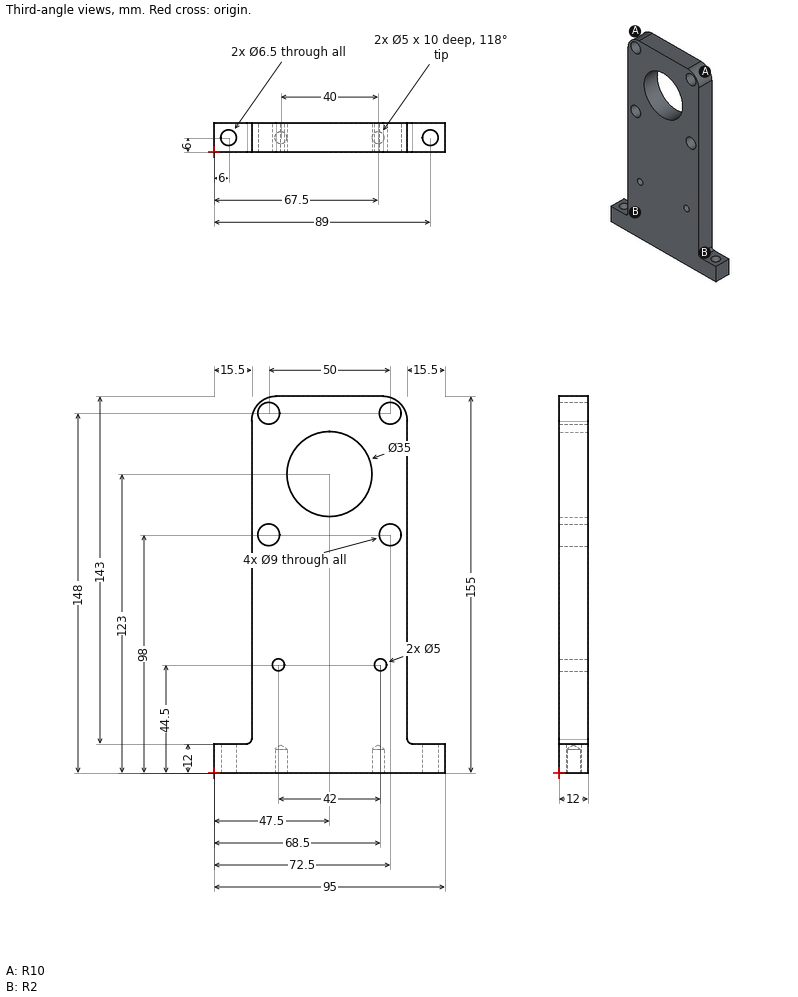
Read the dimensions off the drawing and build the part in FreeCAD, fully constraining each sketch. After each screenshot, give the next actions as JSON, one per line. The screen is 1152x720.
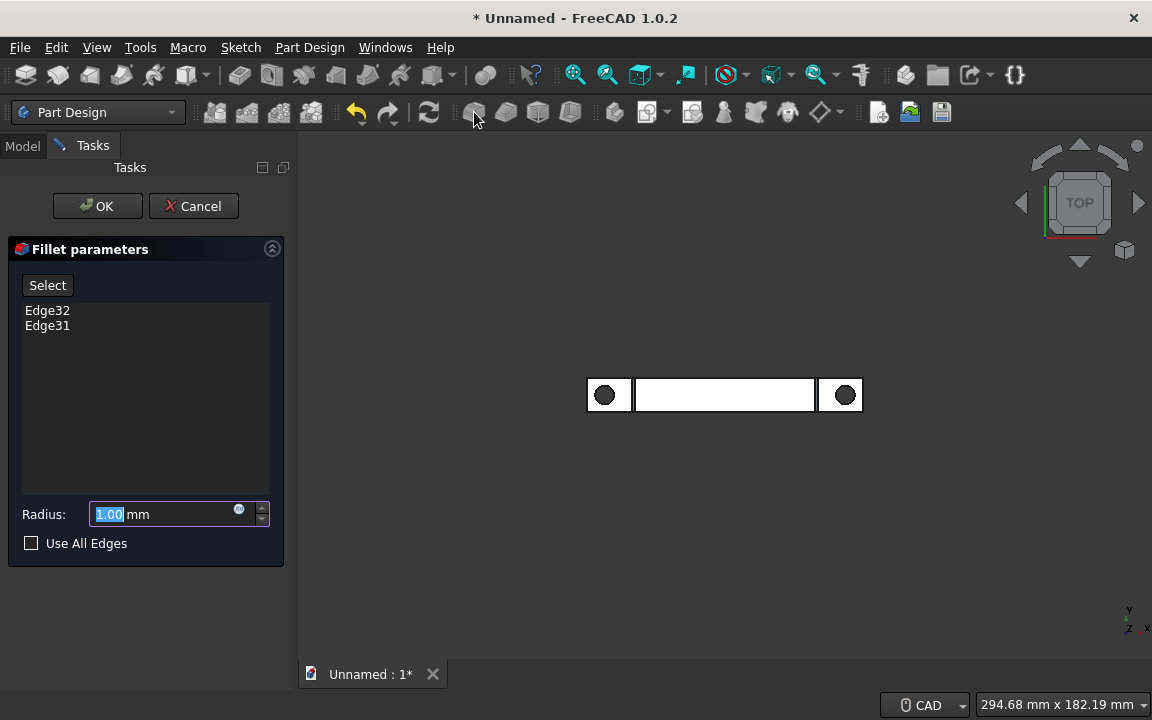
{"action": "type", "text": "10"}
{"action": "key", "text": "Tab"}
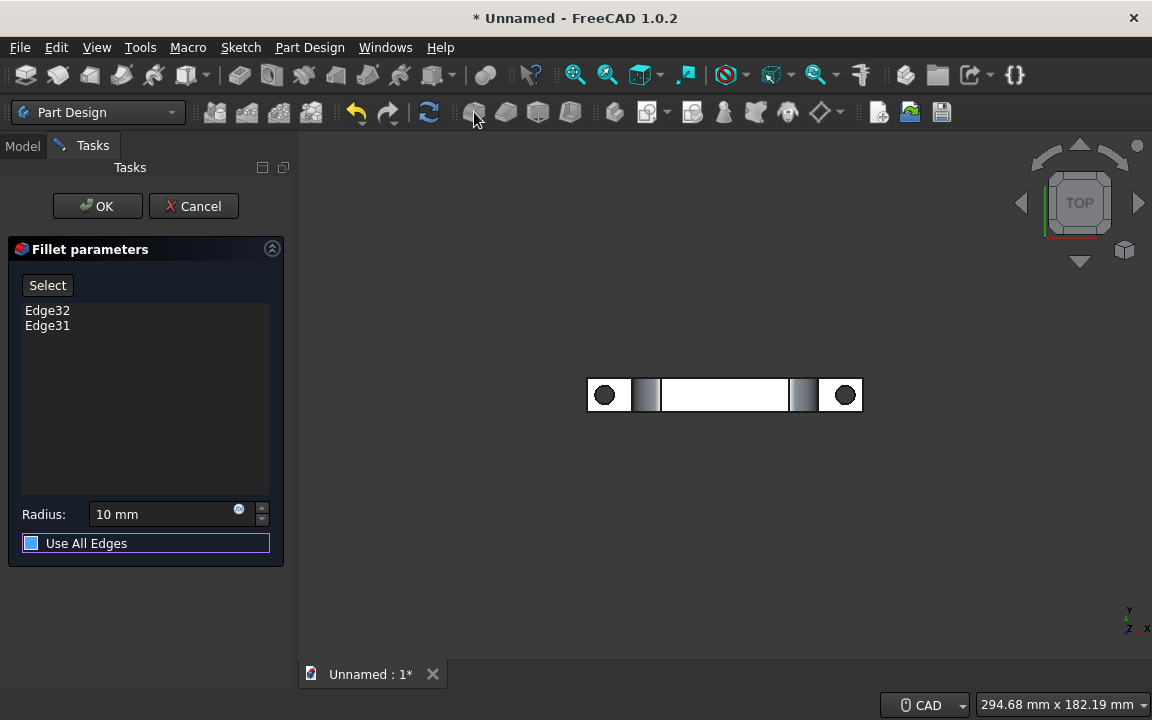
{"action": "left_click", "coordinate": [98, 206]}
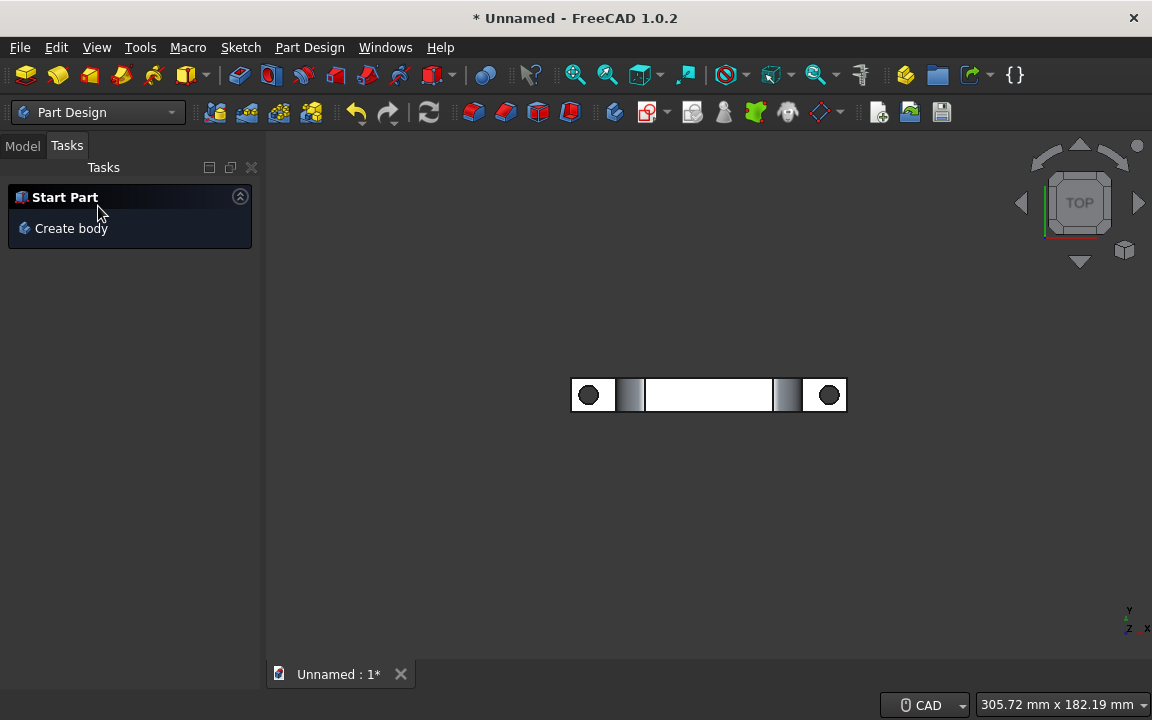
{"action": "left_click", "coordinate": [576, 76]}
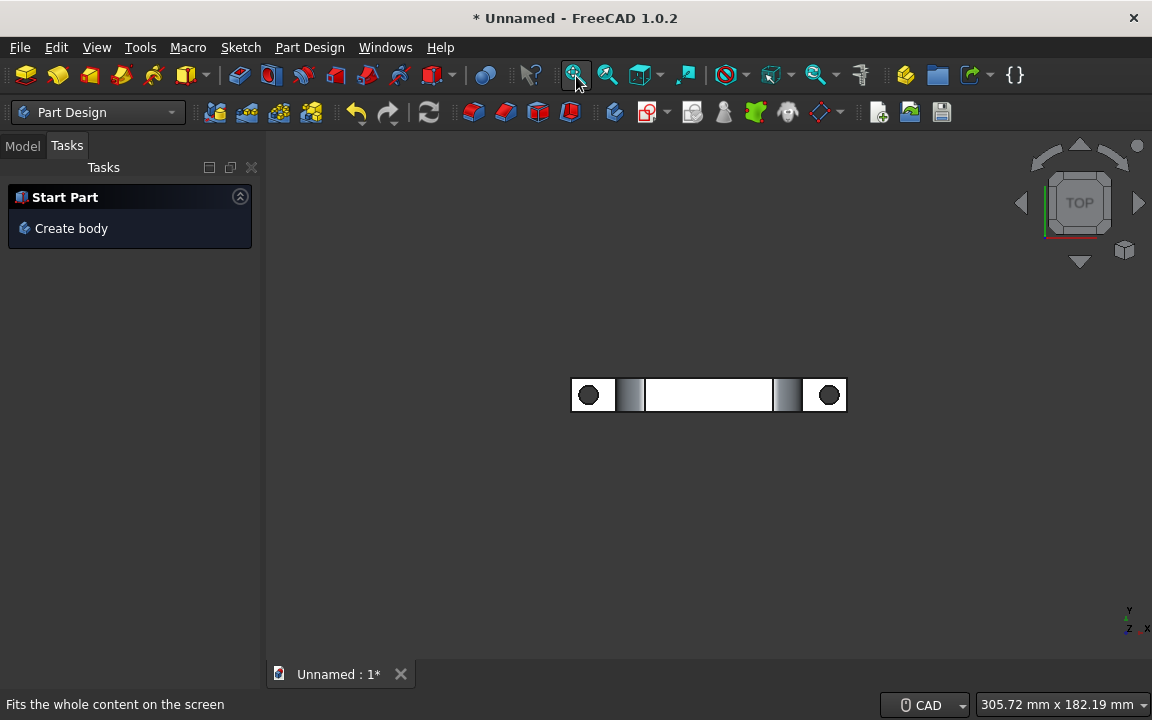
{"action": "key", "text": "5"}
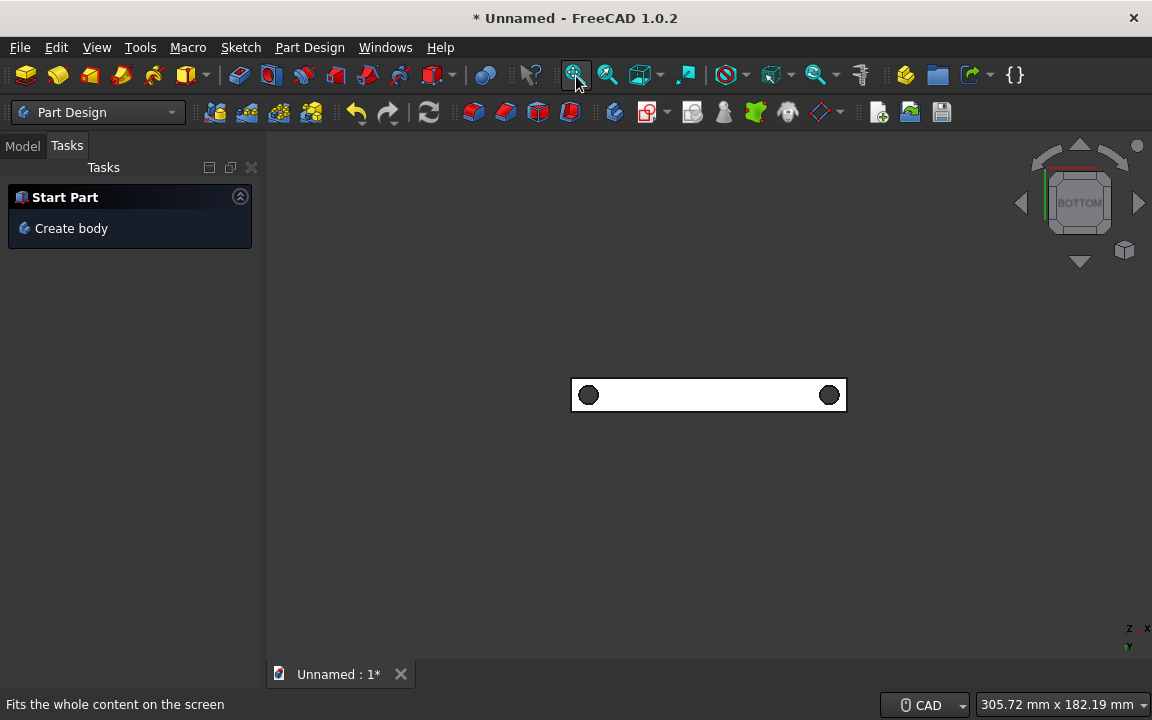
{"action": "left_click", "coordinate": [576, 76]}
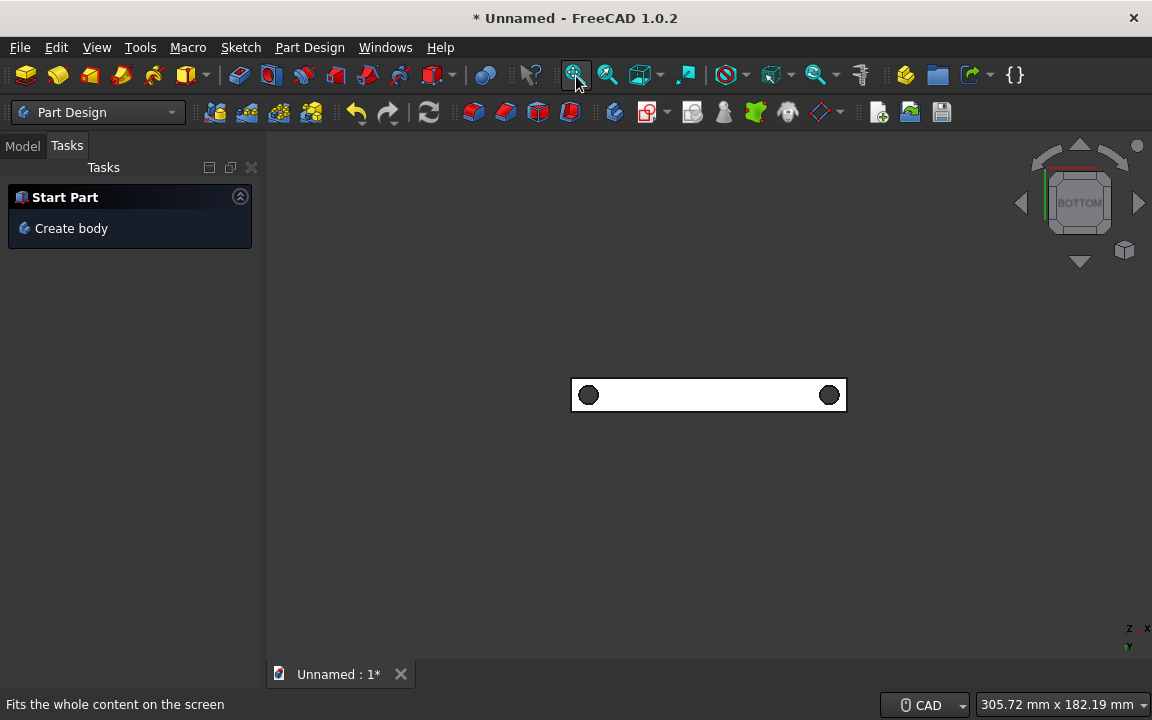
{"action": "left_click", "coordinate": [788, 394]}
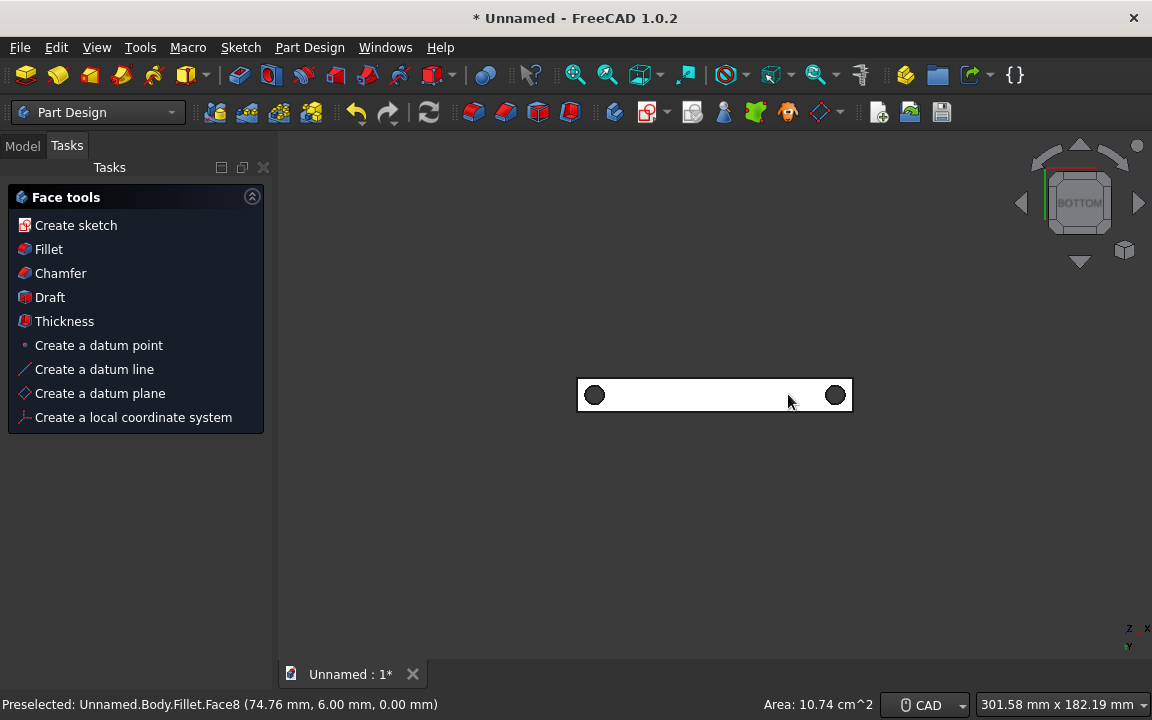
{"action": "left_click", "coordinate": [648, 112]}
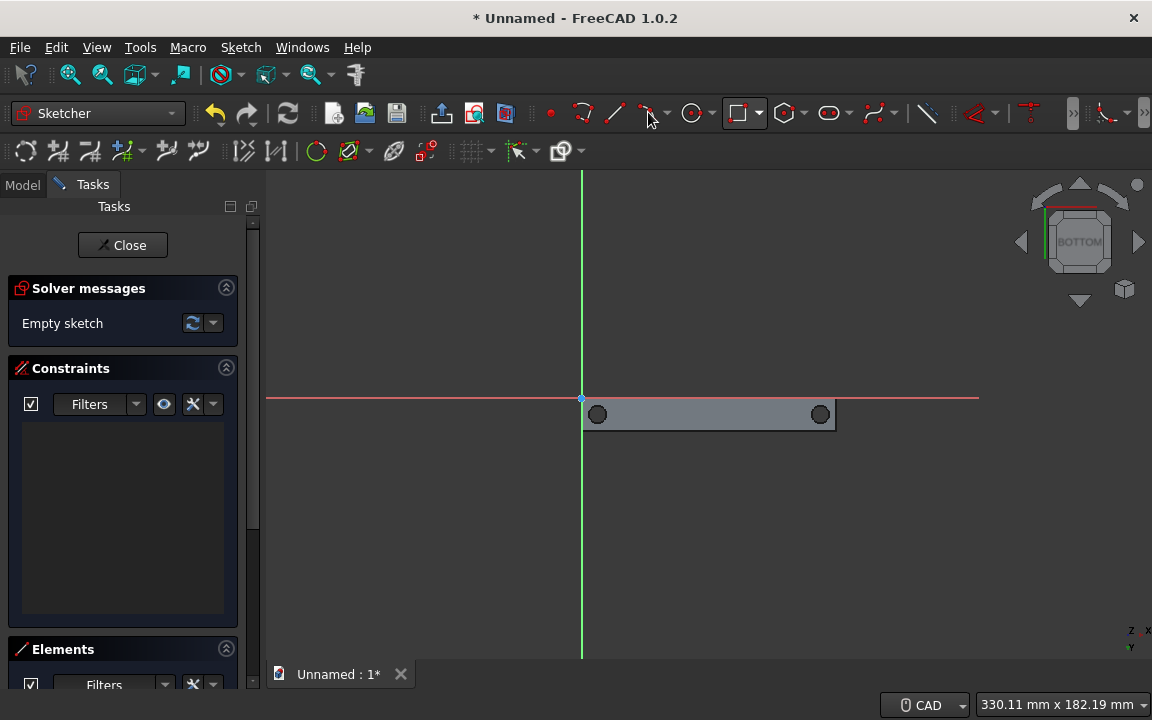
{"action": "scroll", "coordinate": [696, 407], "scroll_direction": "up", "scroll_amount": 5}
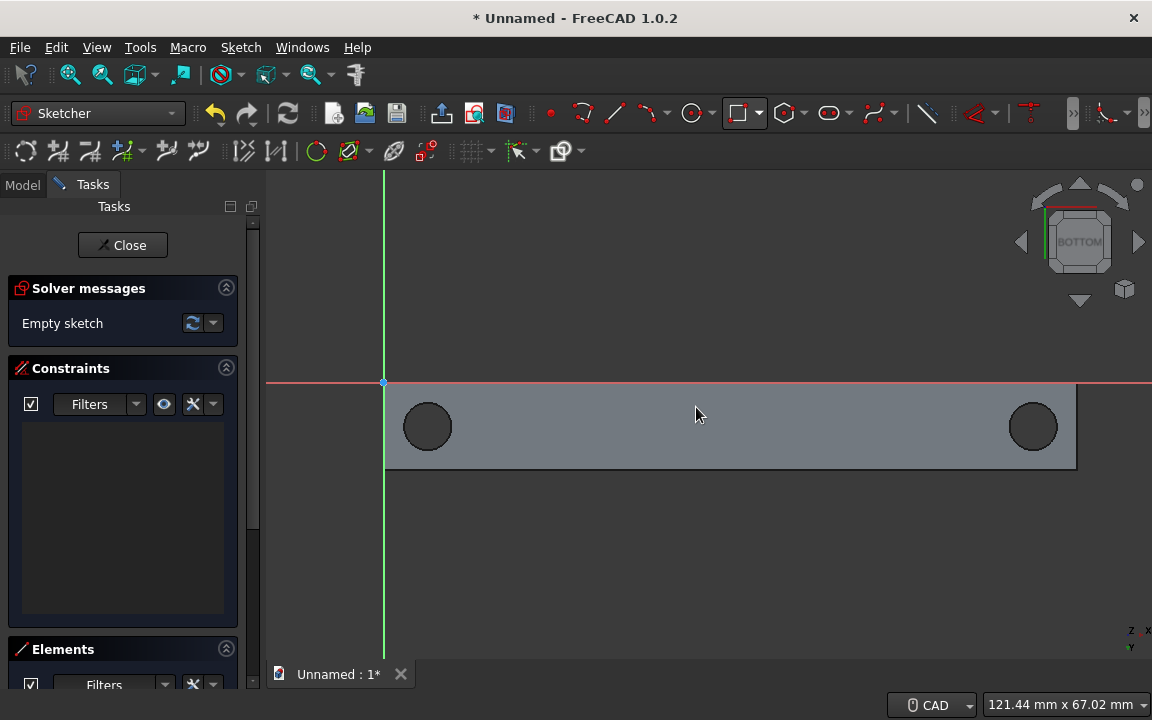
{"action": "left_click", "coordinate": [692, 114]}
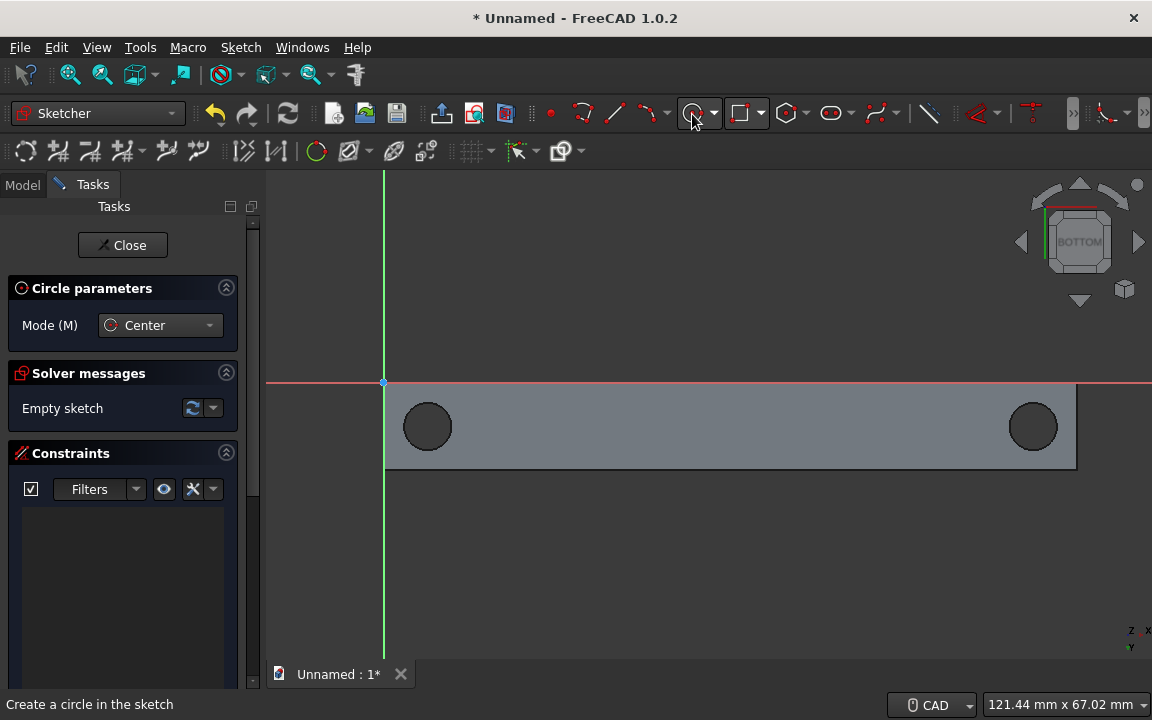
{"action": "scroll", "coordinate": [876, 427], "scroll_direction": "up", "scroll_amount": 2}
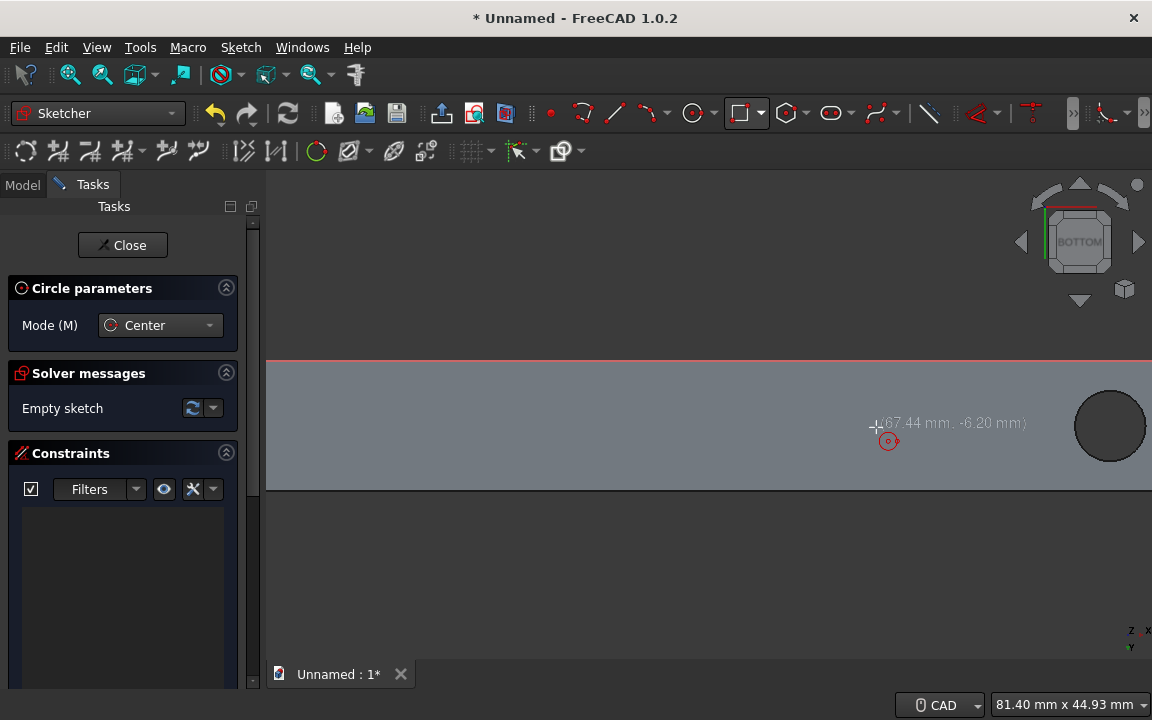
{"action": "left_click", "coordinate": [876, 426]}
{"action": "left_click", "coordinate": [896, 407]}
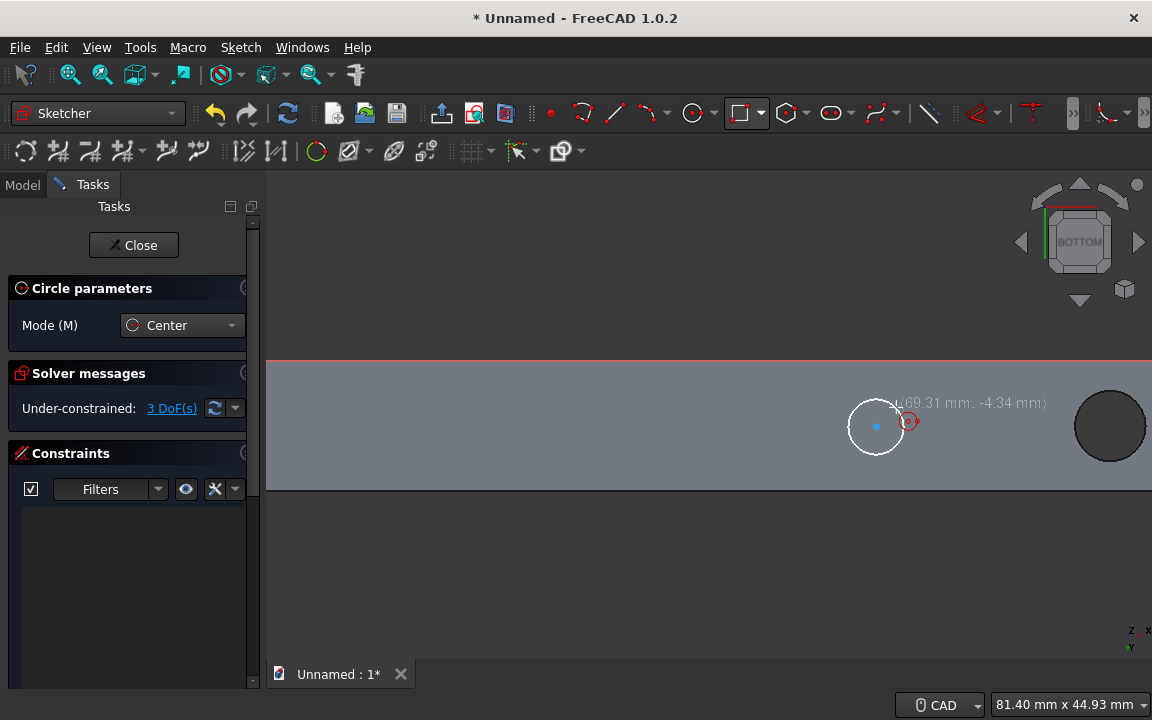
{"action": "left_click", "coordinate": [441, 426]}
{"action": "left_click", "coordinate": [460, 407]}
{"action": "key", "text": "Escape"}